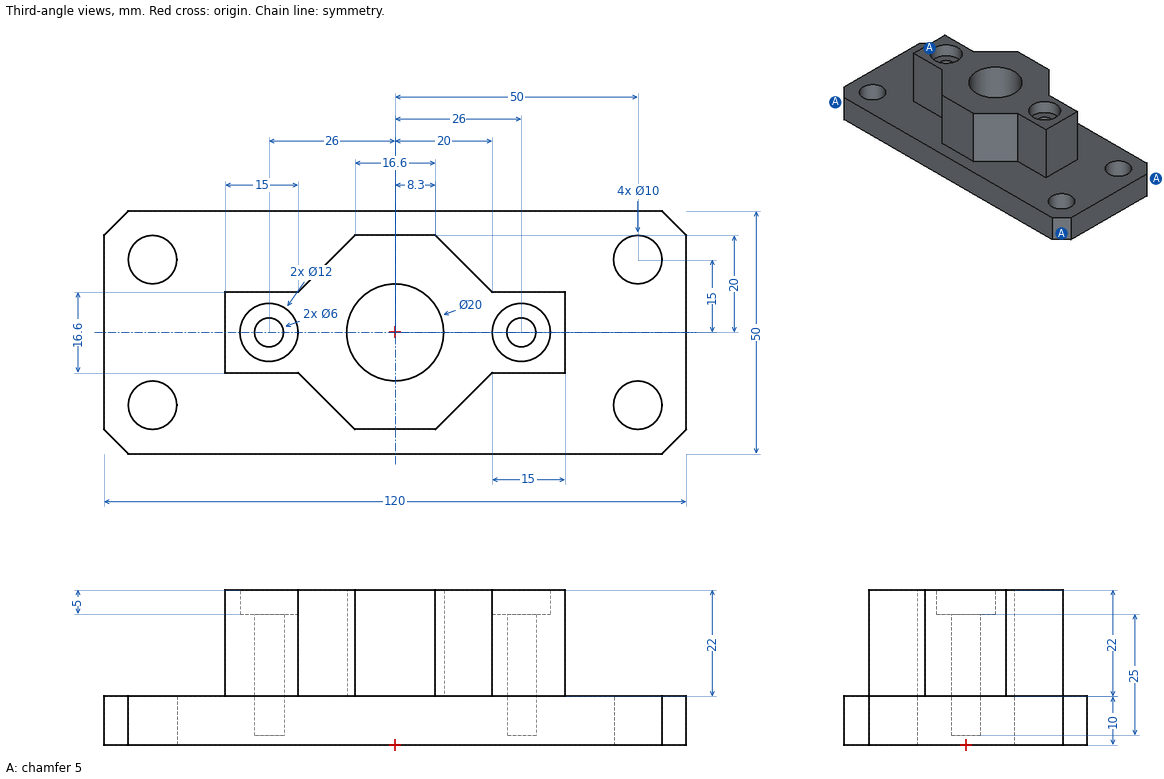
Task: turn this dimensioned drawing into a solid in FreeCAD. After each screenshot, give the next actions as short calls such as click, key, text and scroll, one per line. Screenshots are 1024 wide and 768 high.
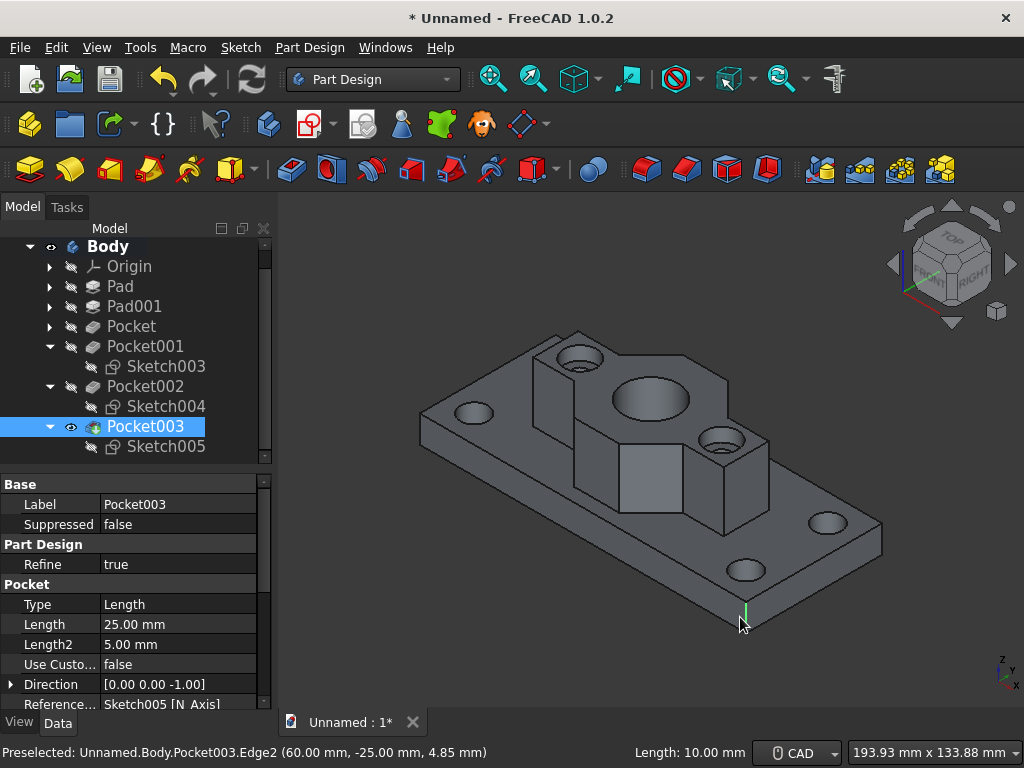
key(2)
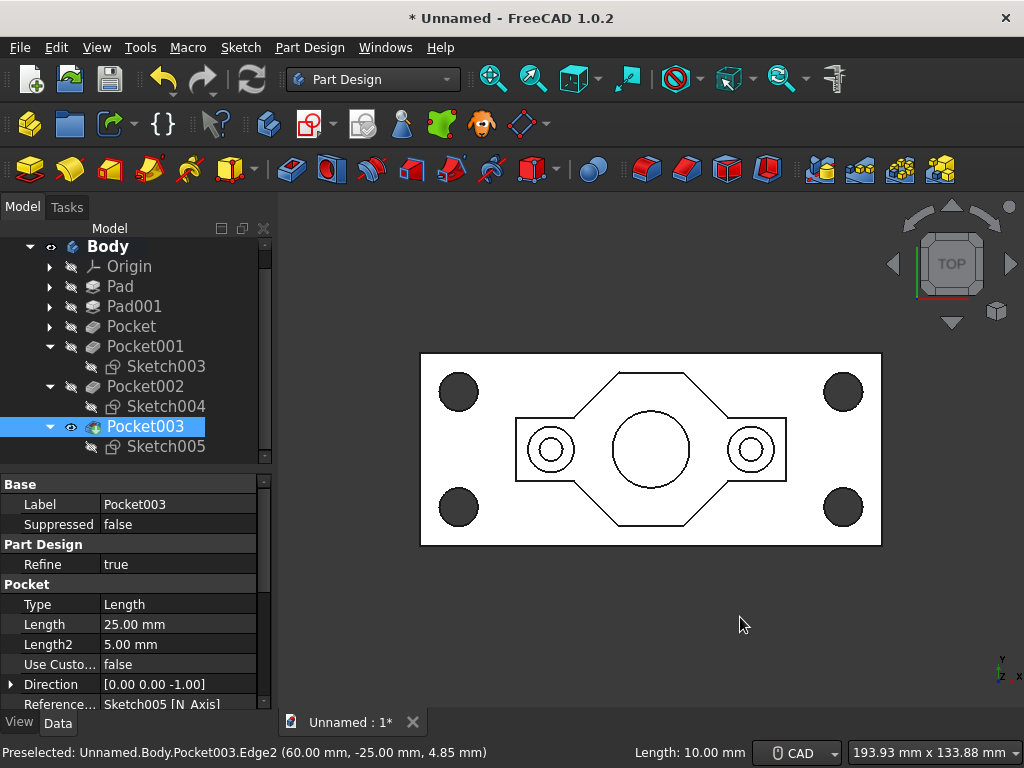
key(1)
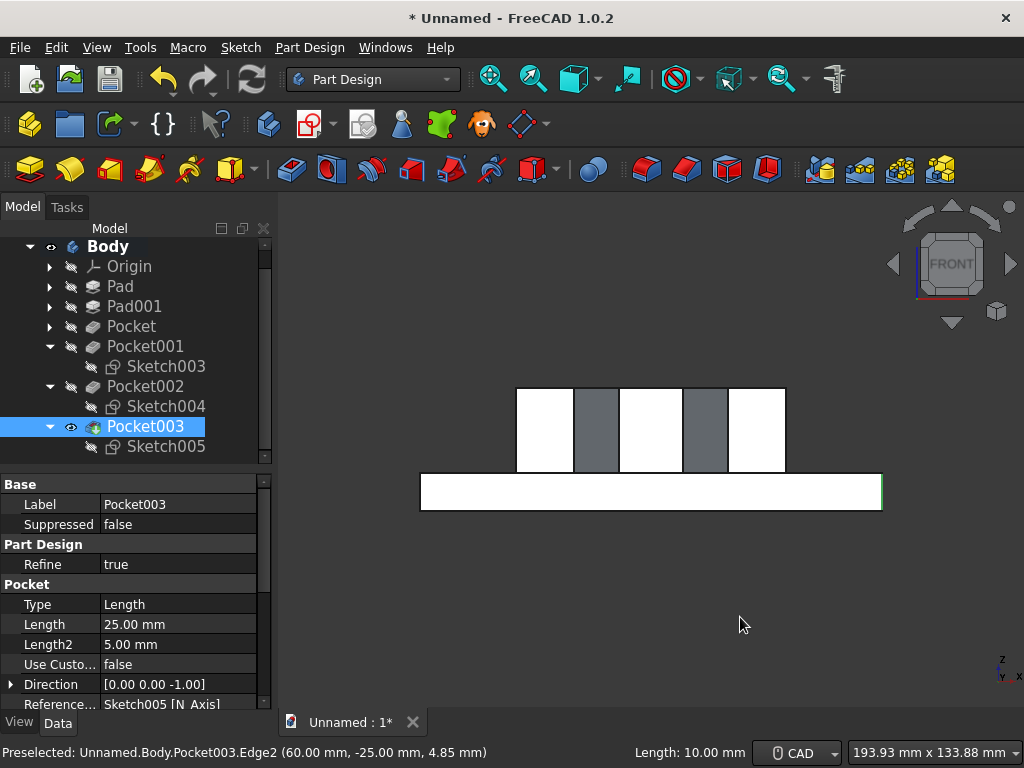
click(420, 491, ctrl)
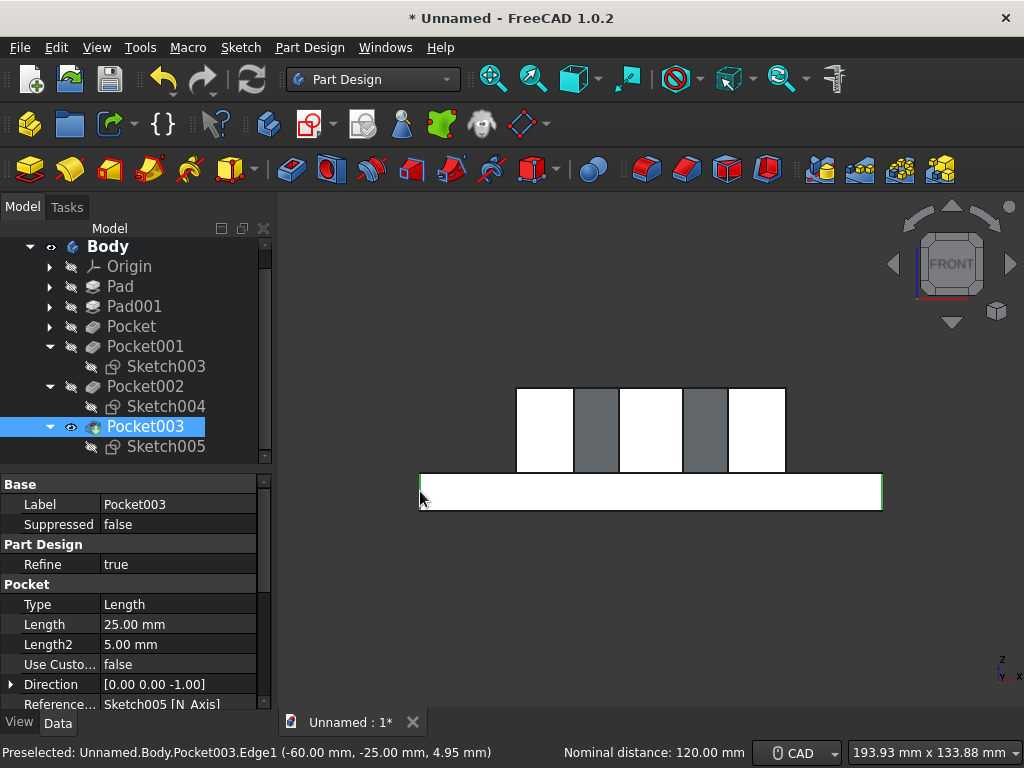
key(3)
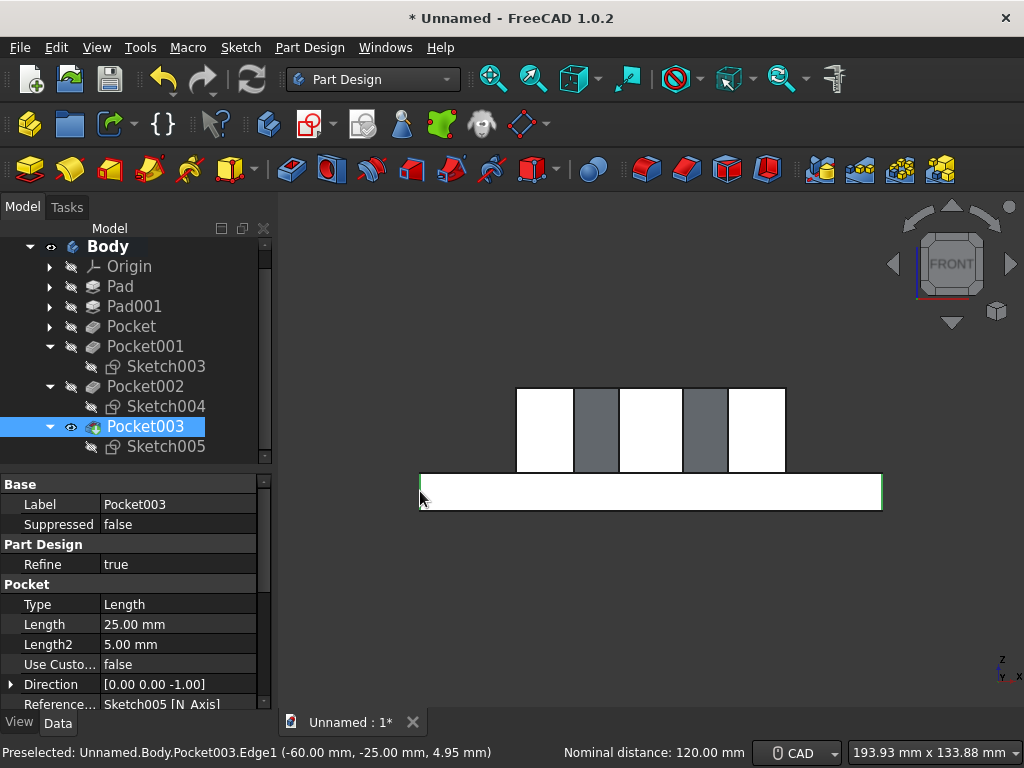
key(v)
key(f)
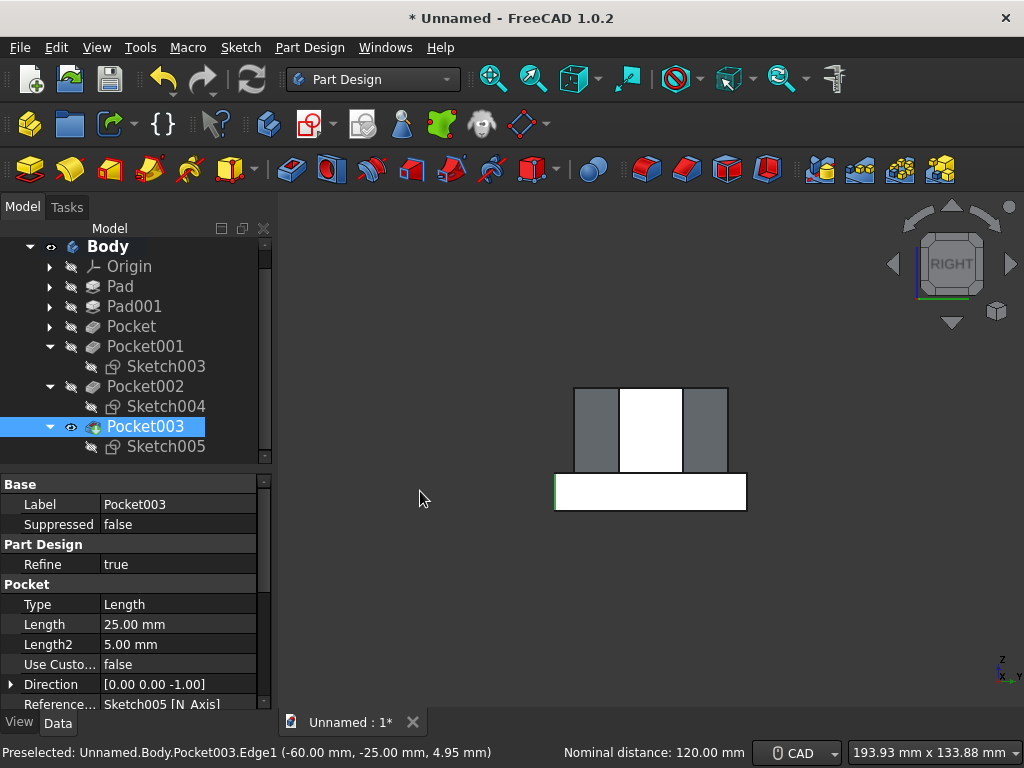
click(747, 491, ctrl)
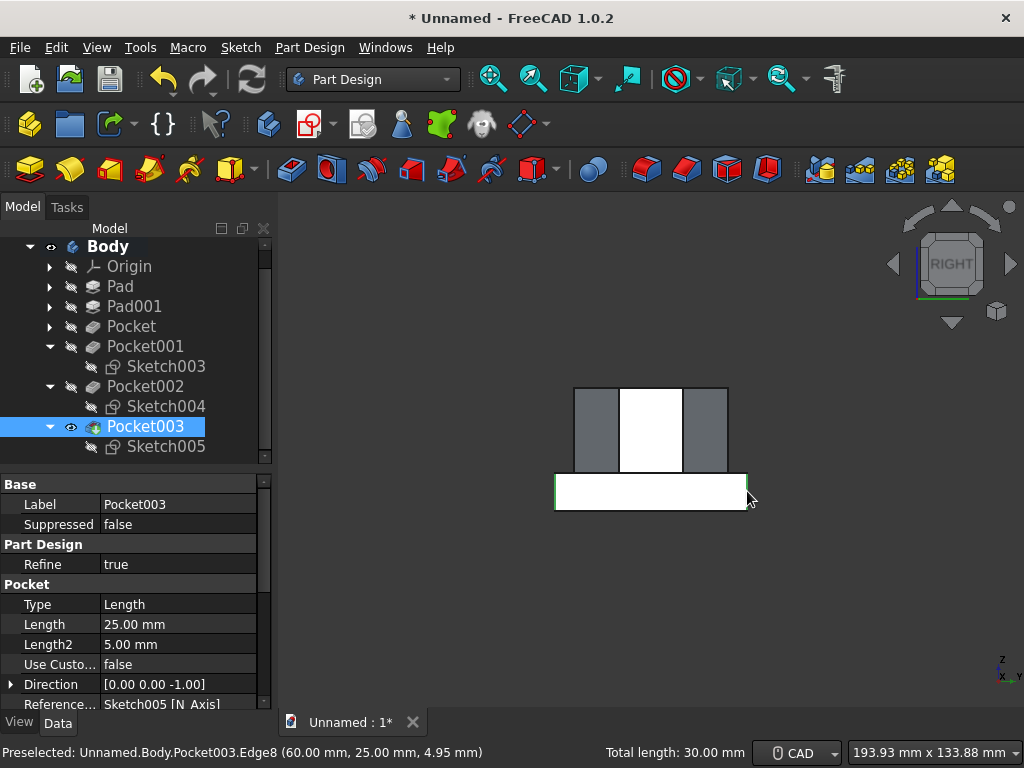
key(5)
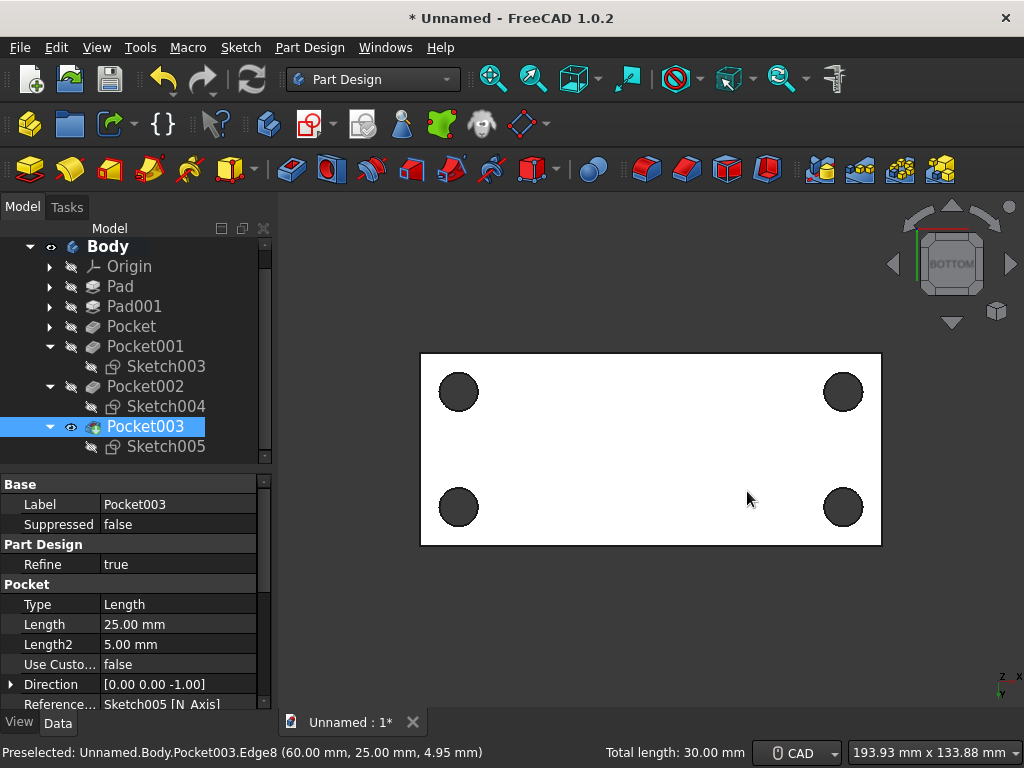
key(4)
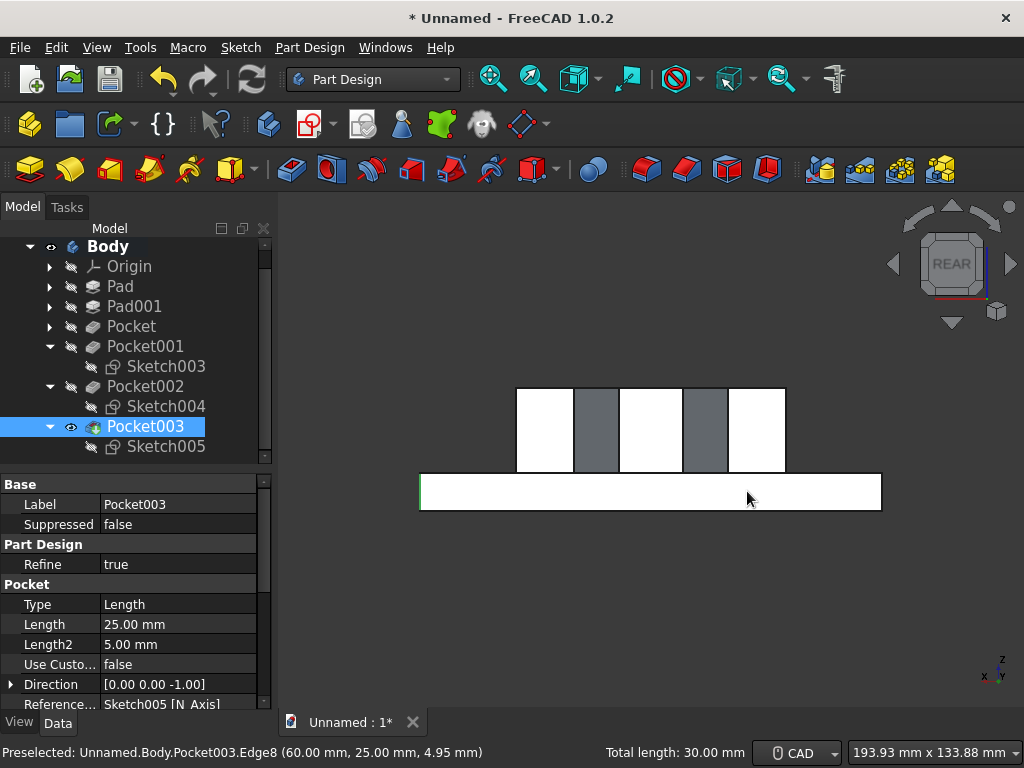
click(882, 491, ctrl)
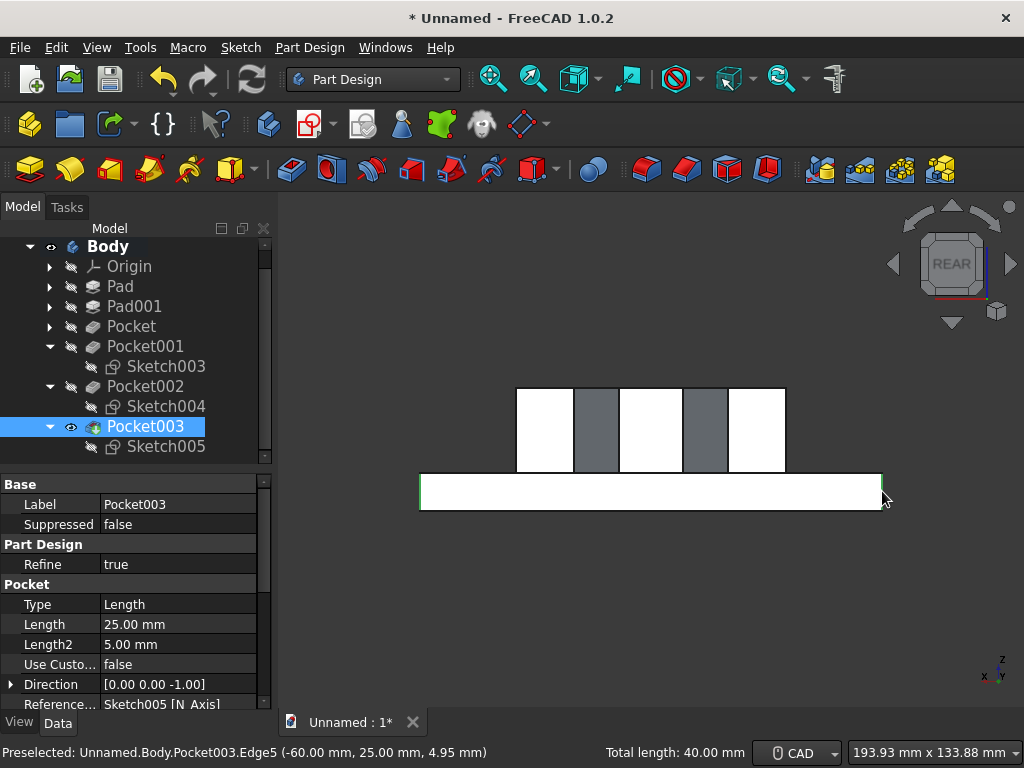
click(688, 170)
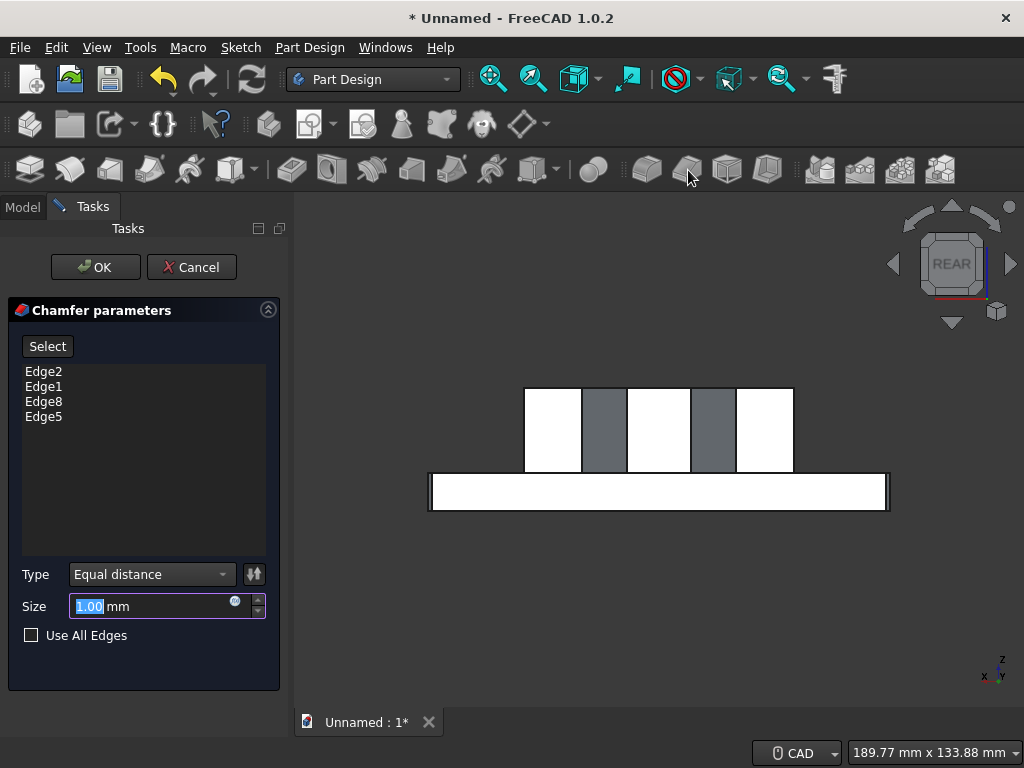
text(5)
key(Tab)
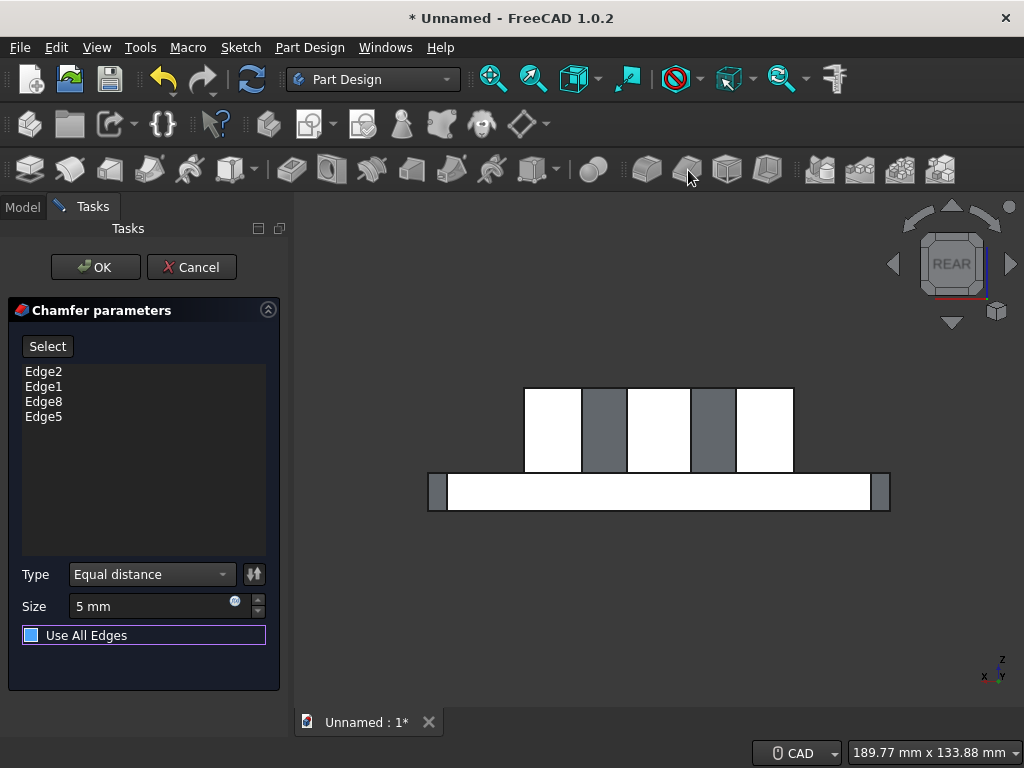
click(96, 267)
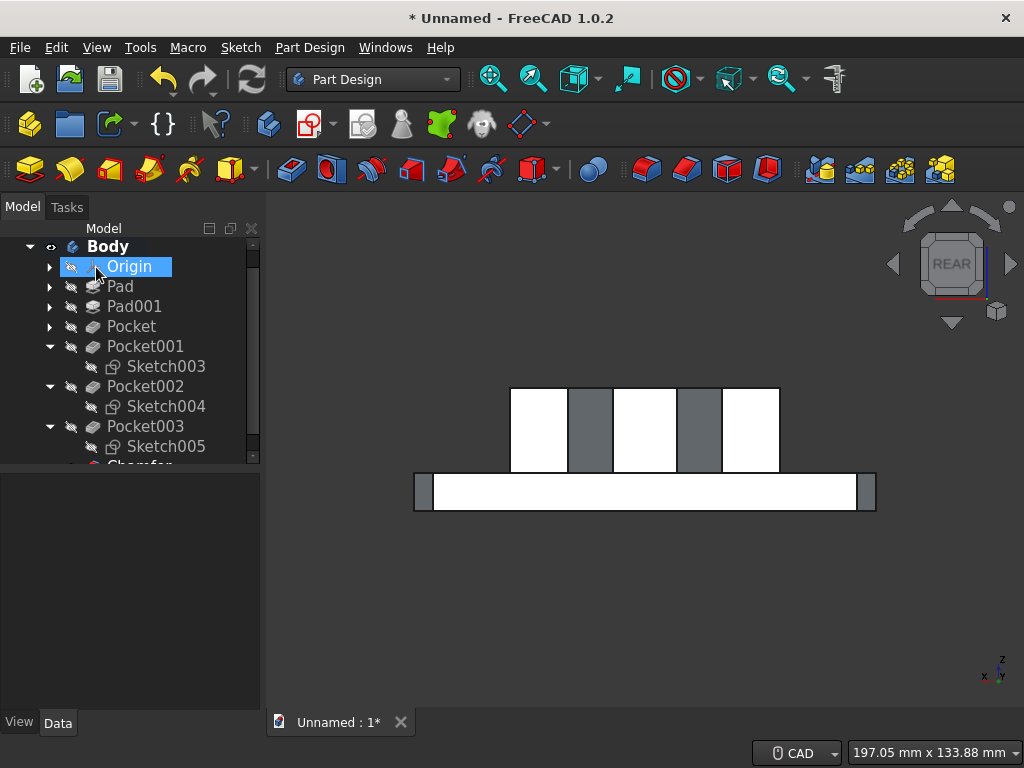
key(0)